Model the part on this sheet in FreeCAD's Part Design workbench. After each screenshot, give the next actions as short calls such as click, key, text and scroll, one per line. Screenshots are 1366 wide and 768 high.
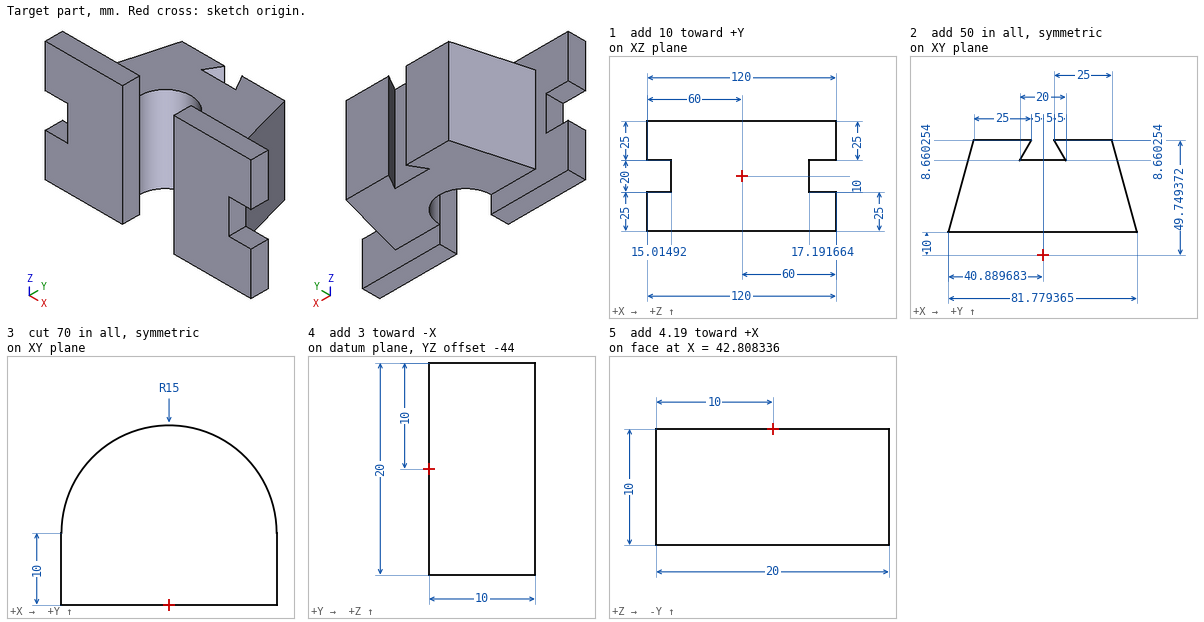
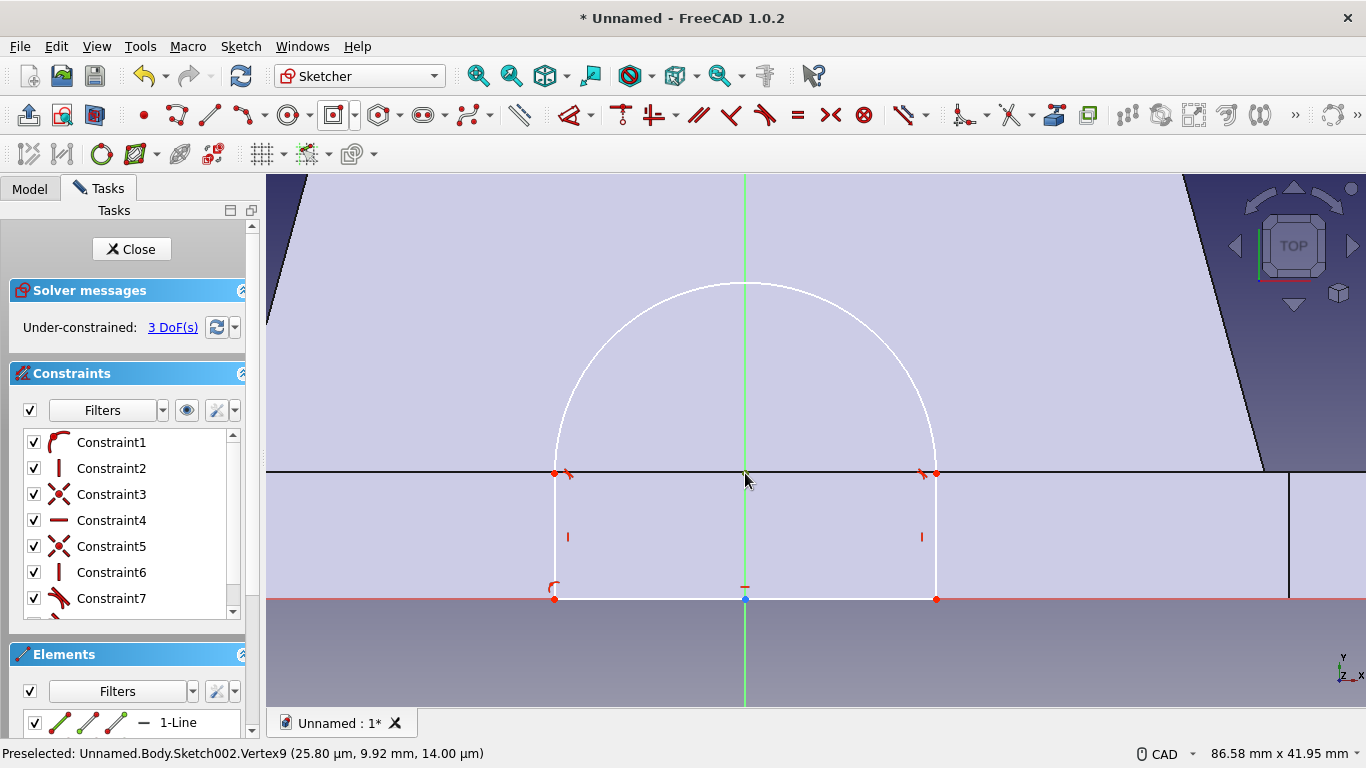
click(745, 645)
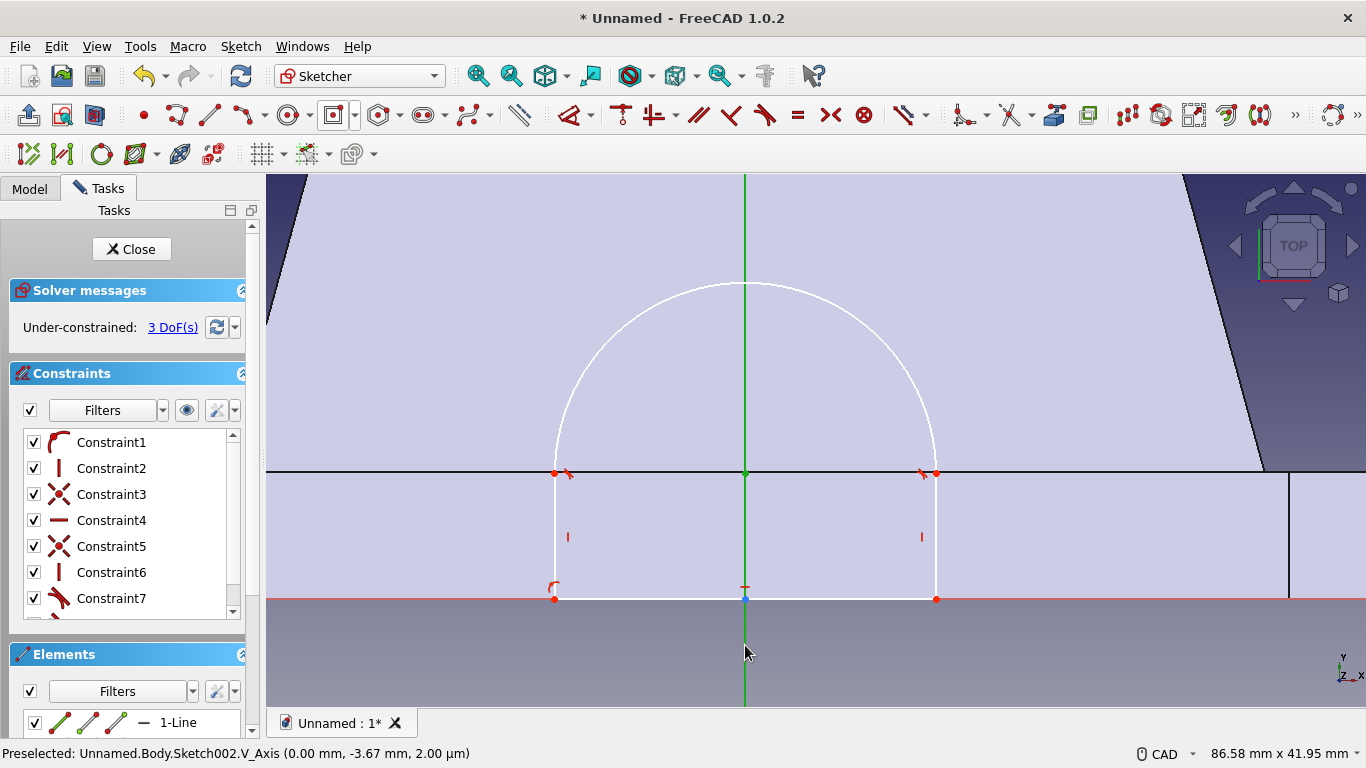
key(c)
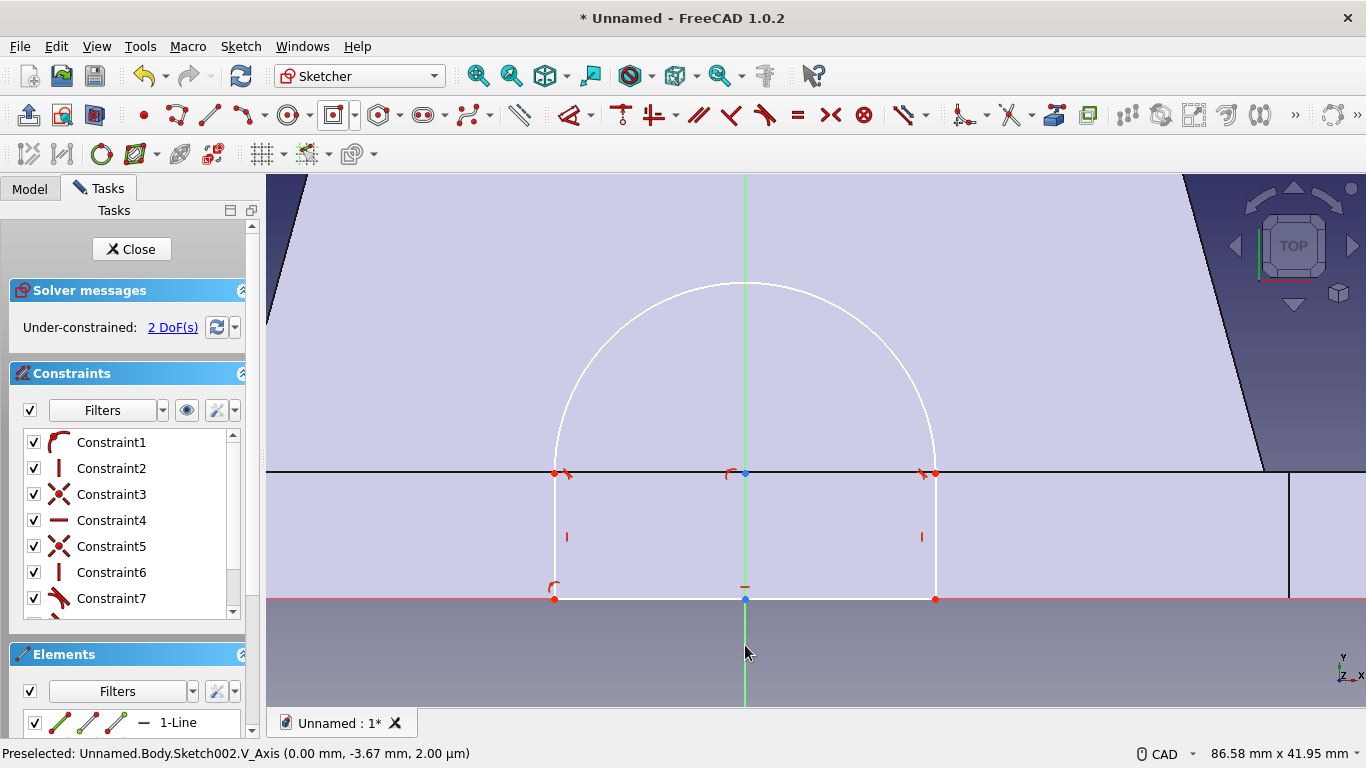
key(d)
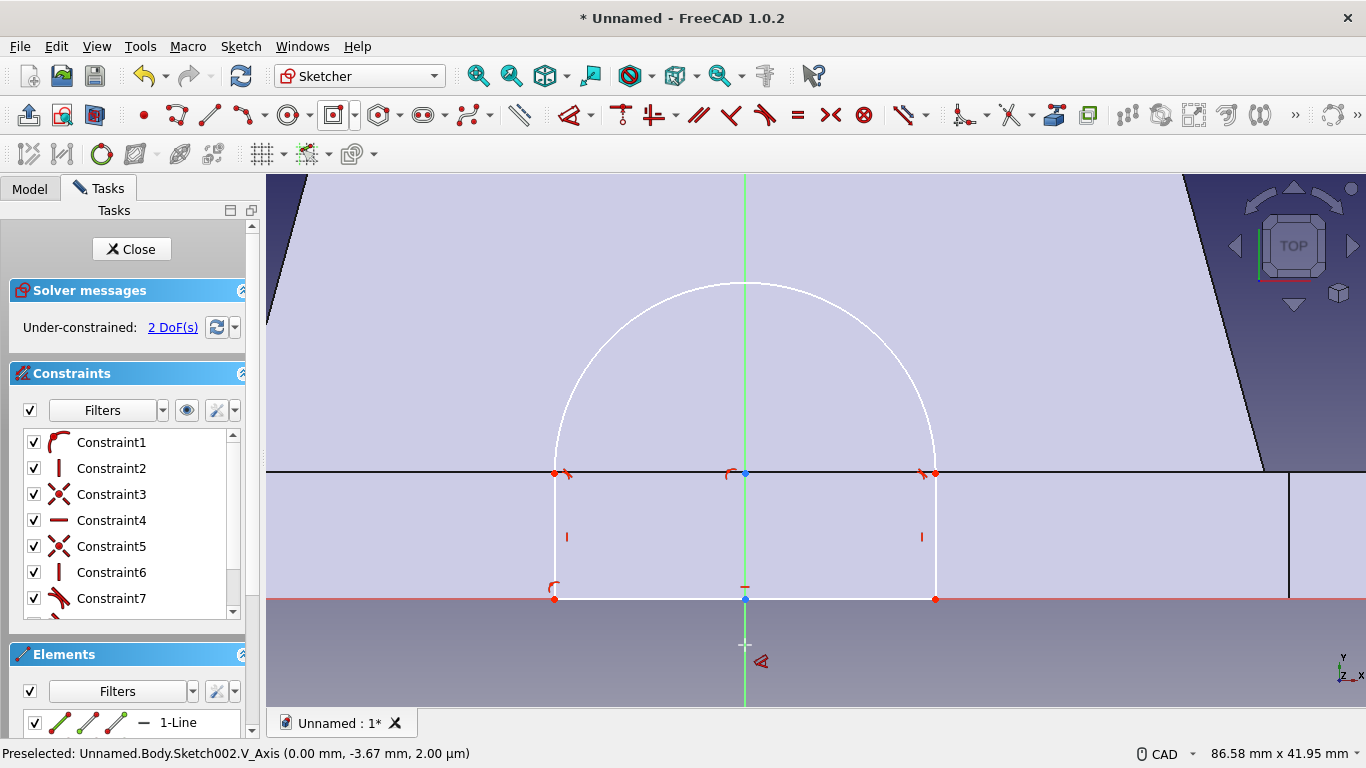
click(857, 319)
click(876, 293)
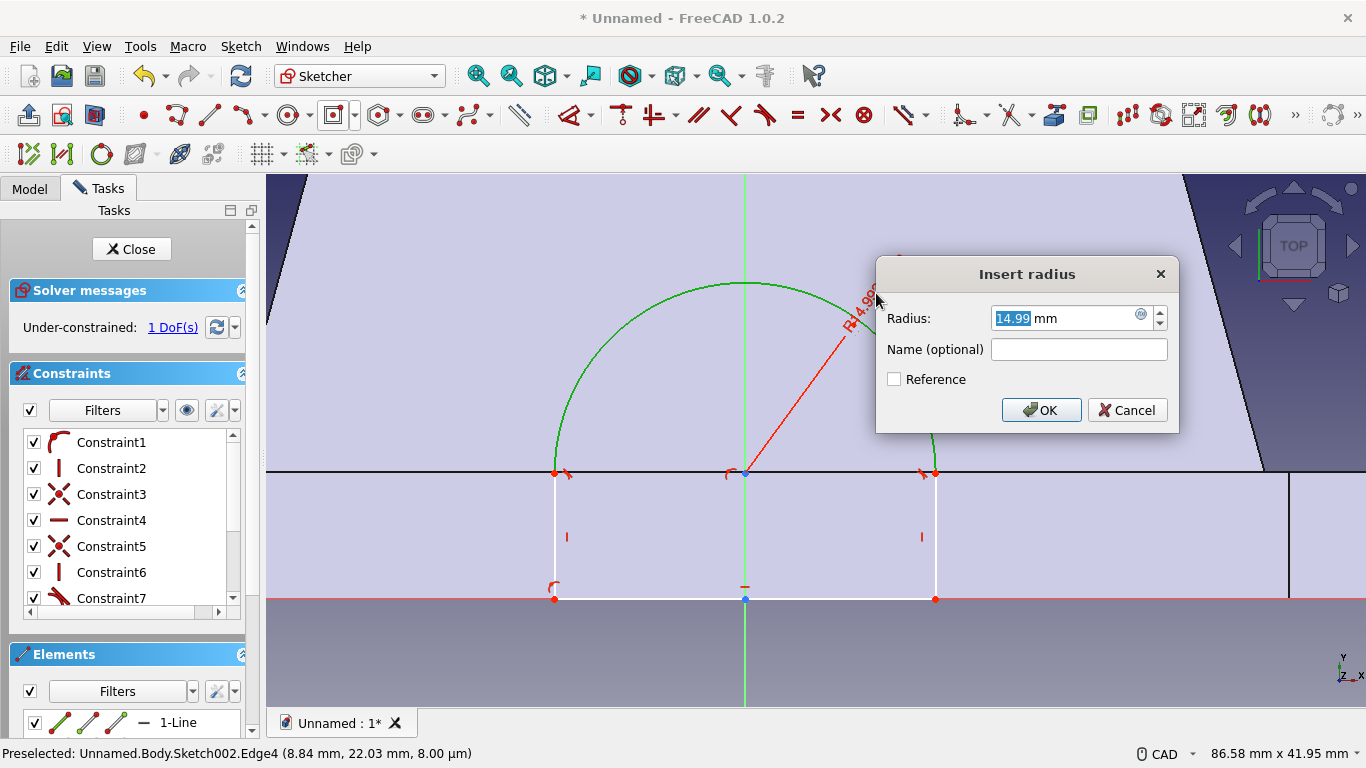
text(15)
key(Return)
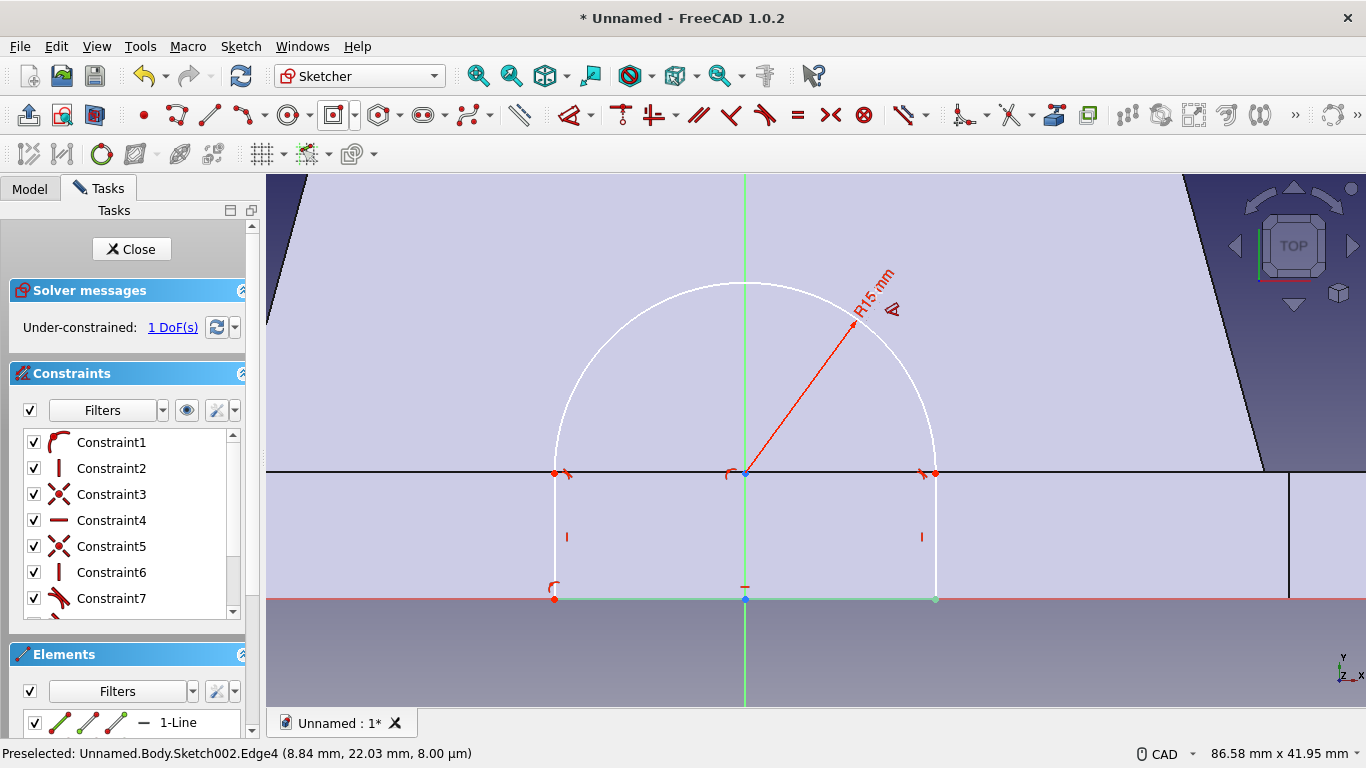
click(555, 511)
click(521, 536)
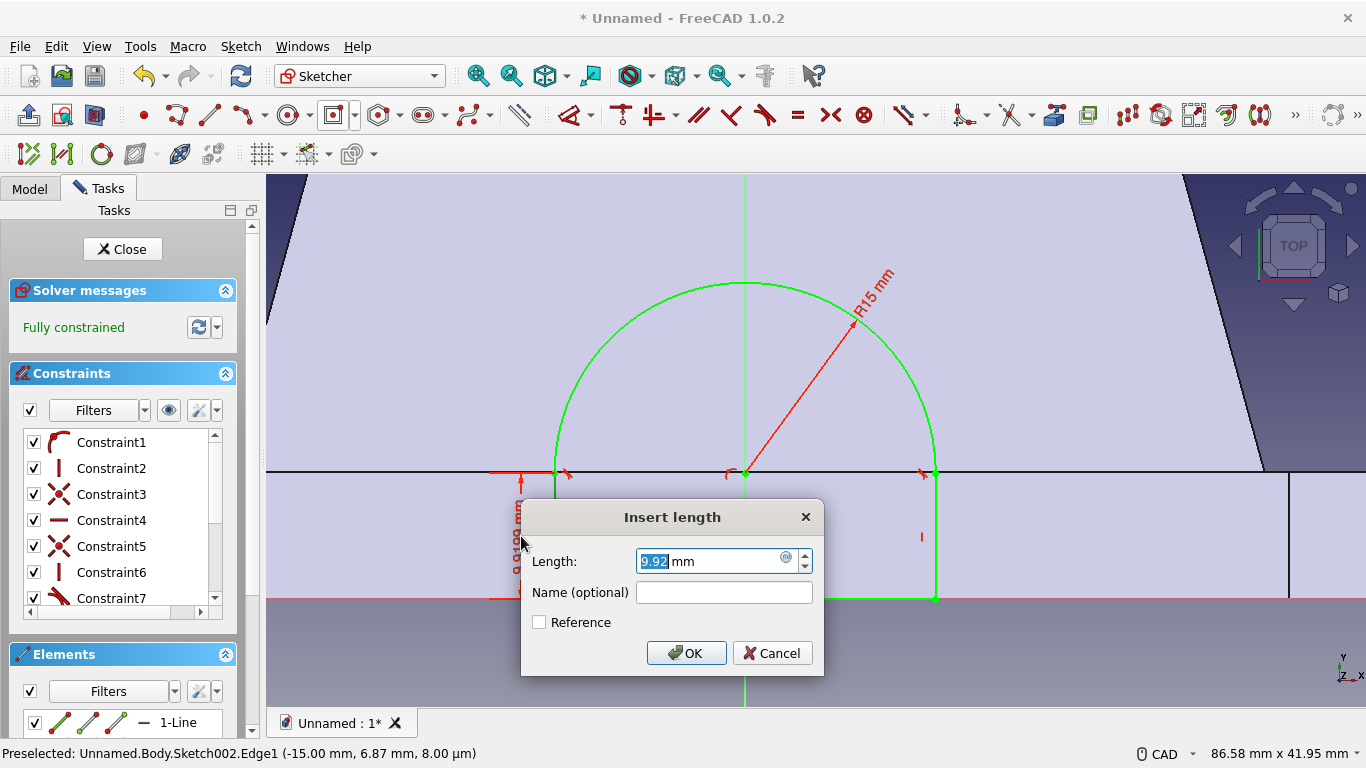
text(10)
key(Return)
key(Escape)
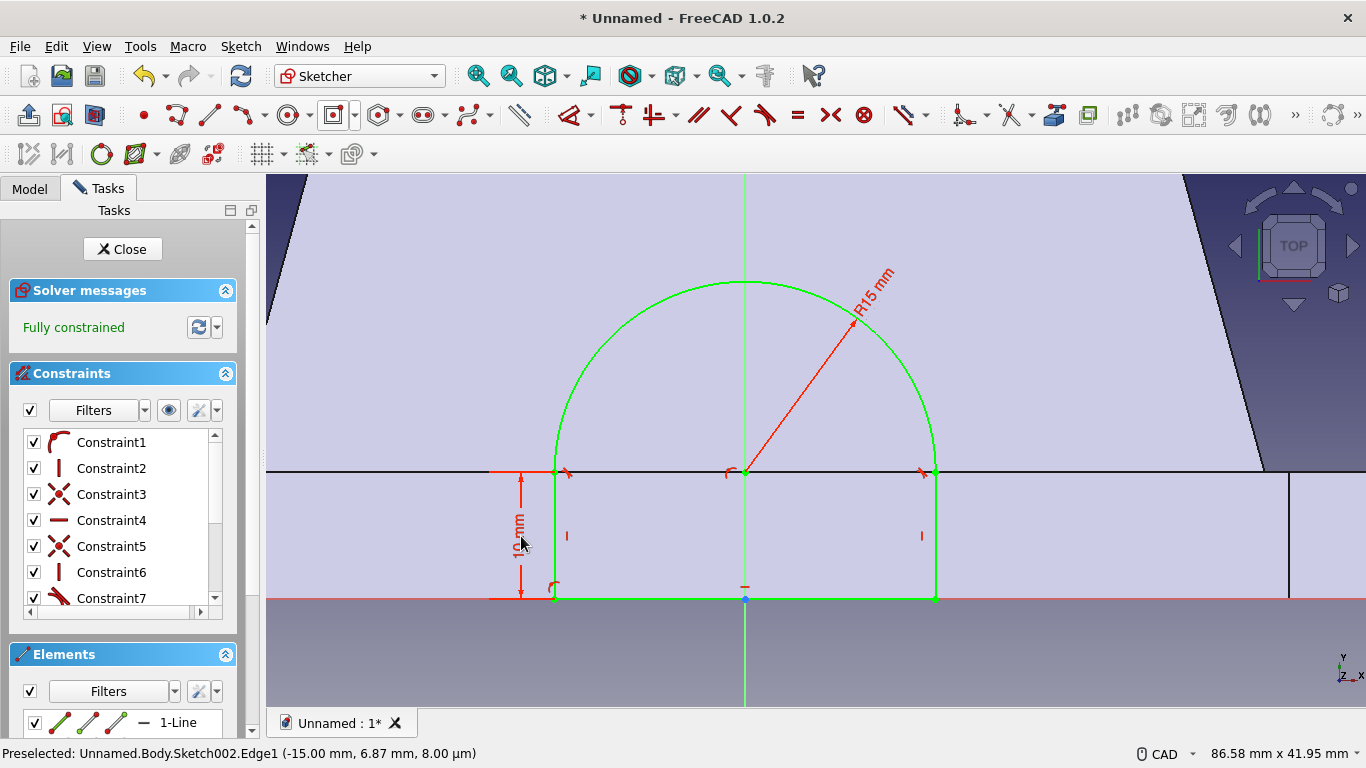
click(123, 249)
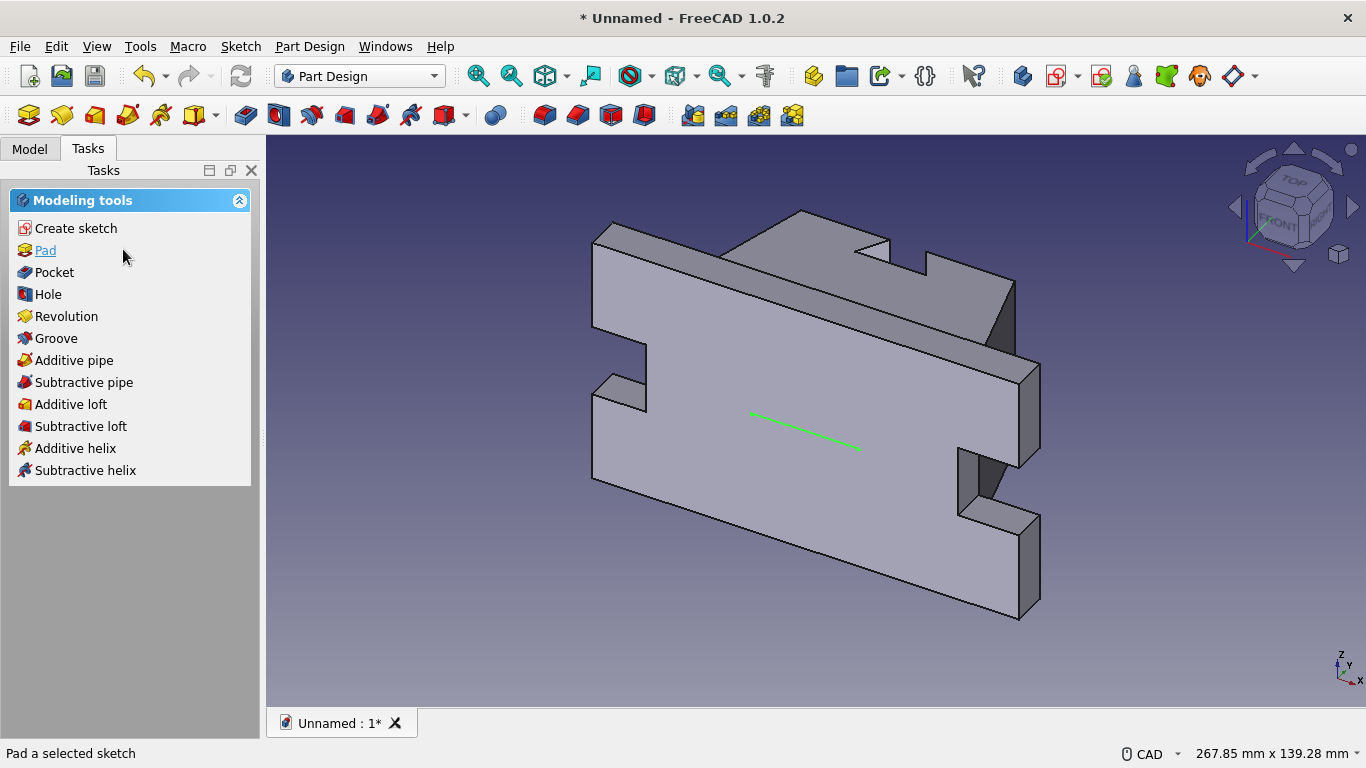
click(246, 116)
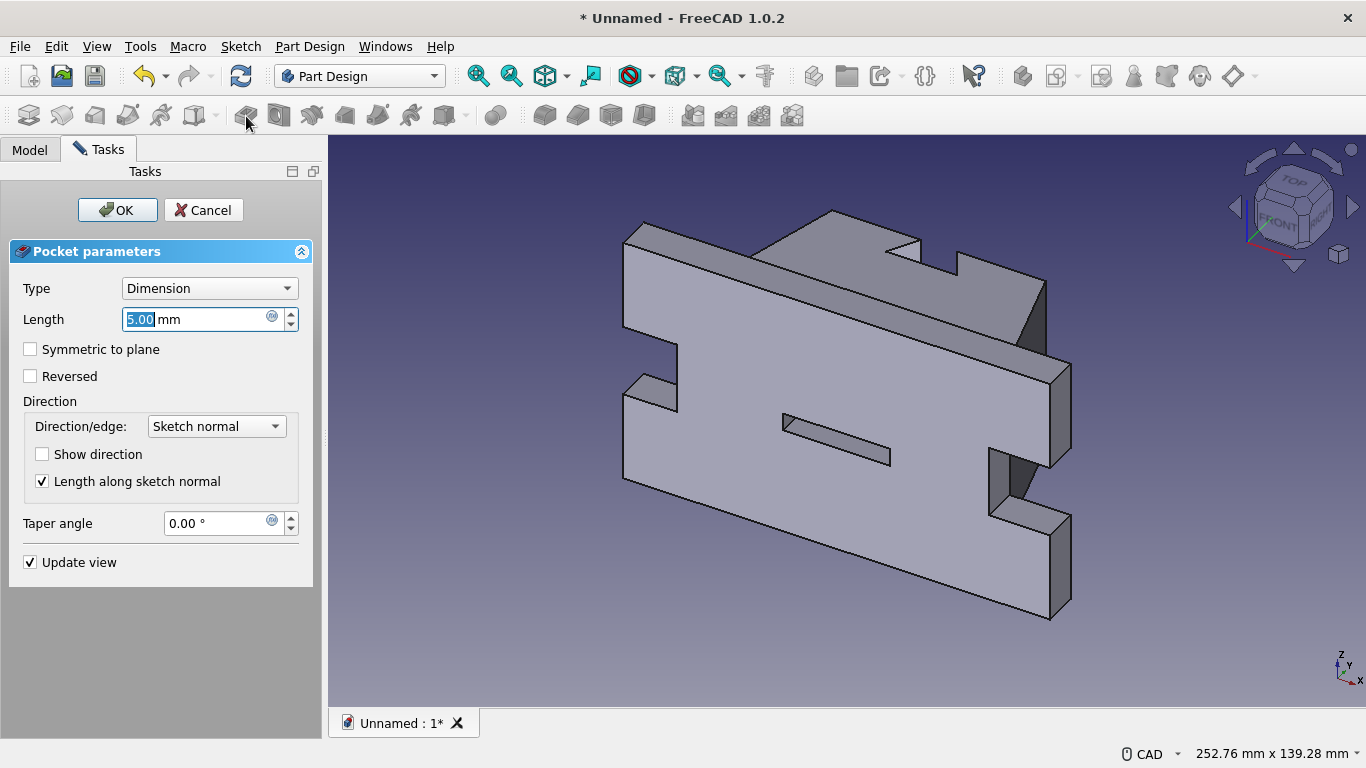
text(70)
key(Tab)